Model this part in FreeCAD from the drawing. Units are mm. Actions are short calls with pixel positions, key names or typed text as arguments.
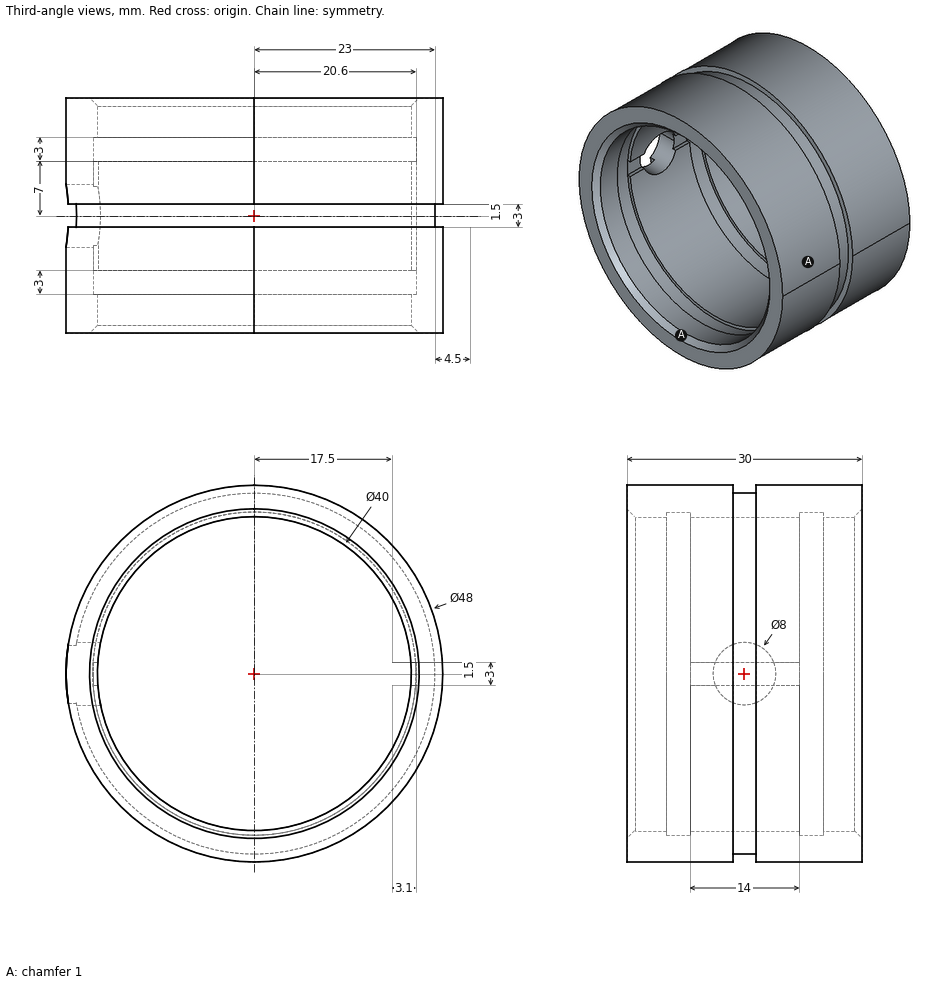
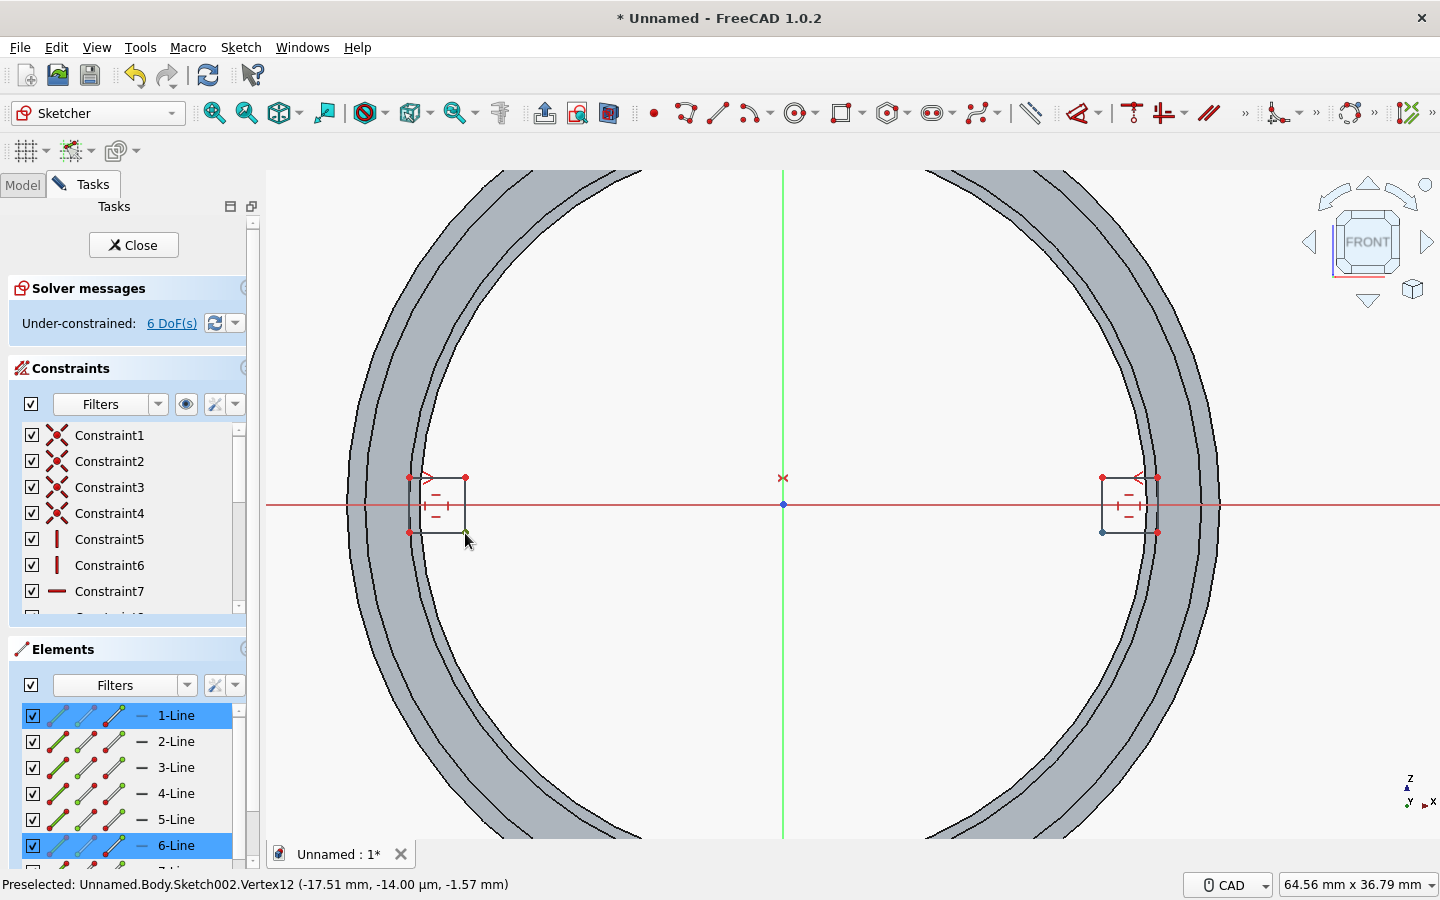
click(783, 767)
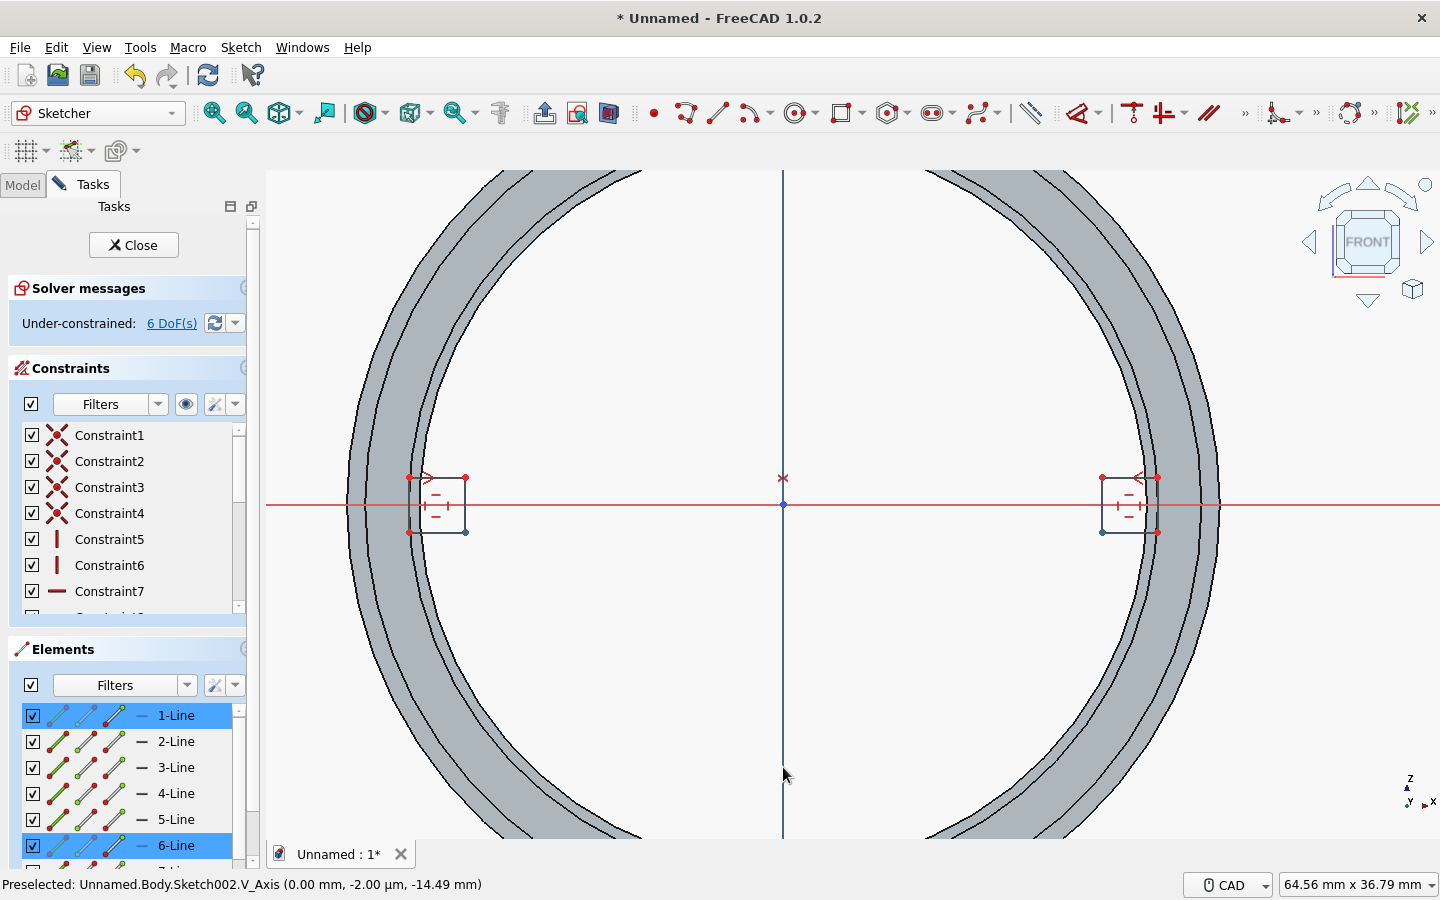
key(s)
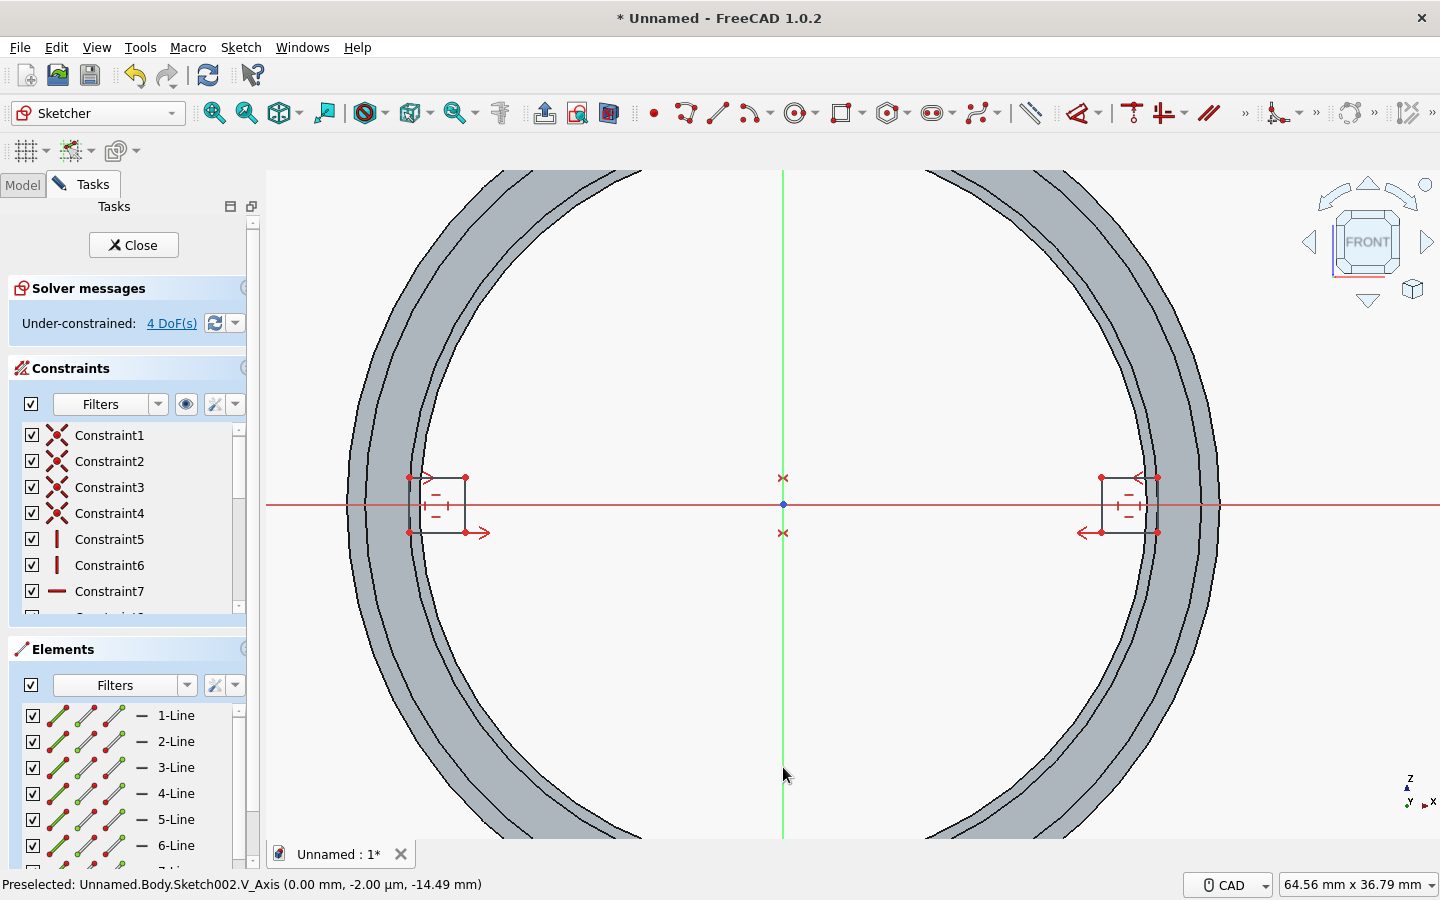
key(d)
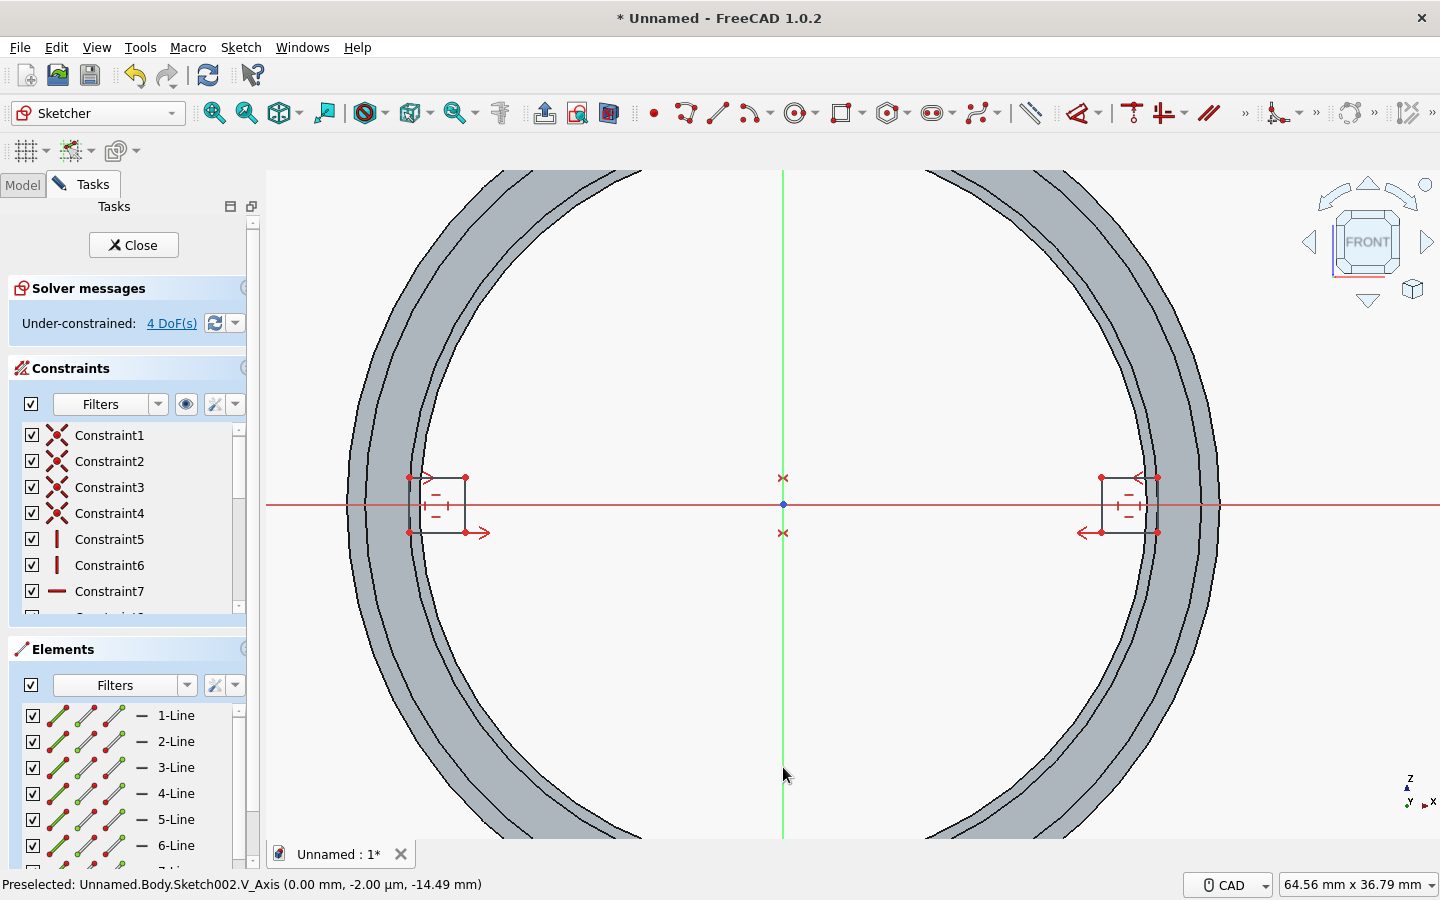
scroll(1102, 495, up, 2)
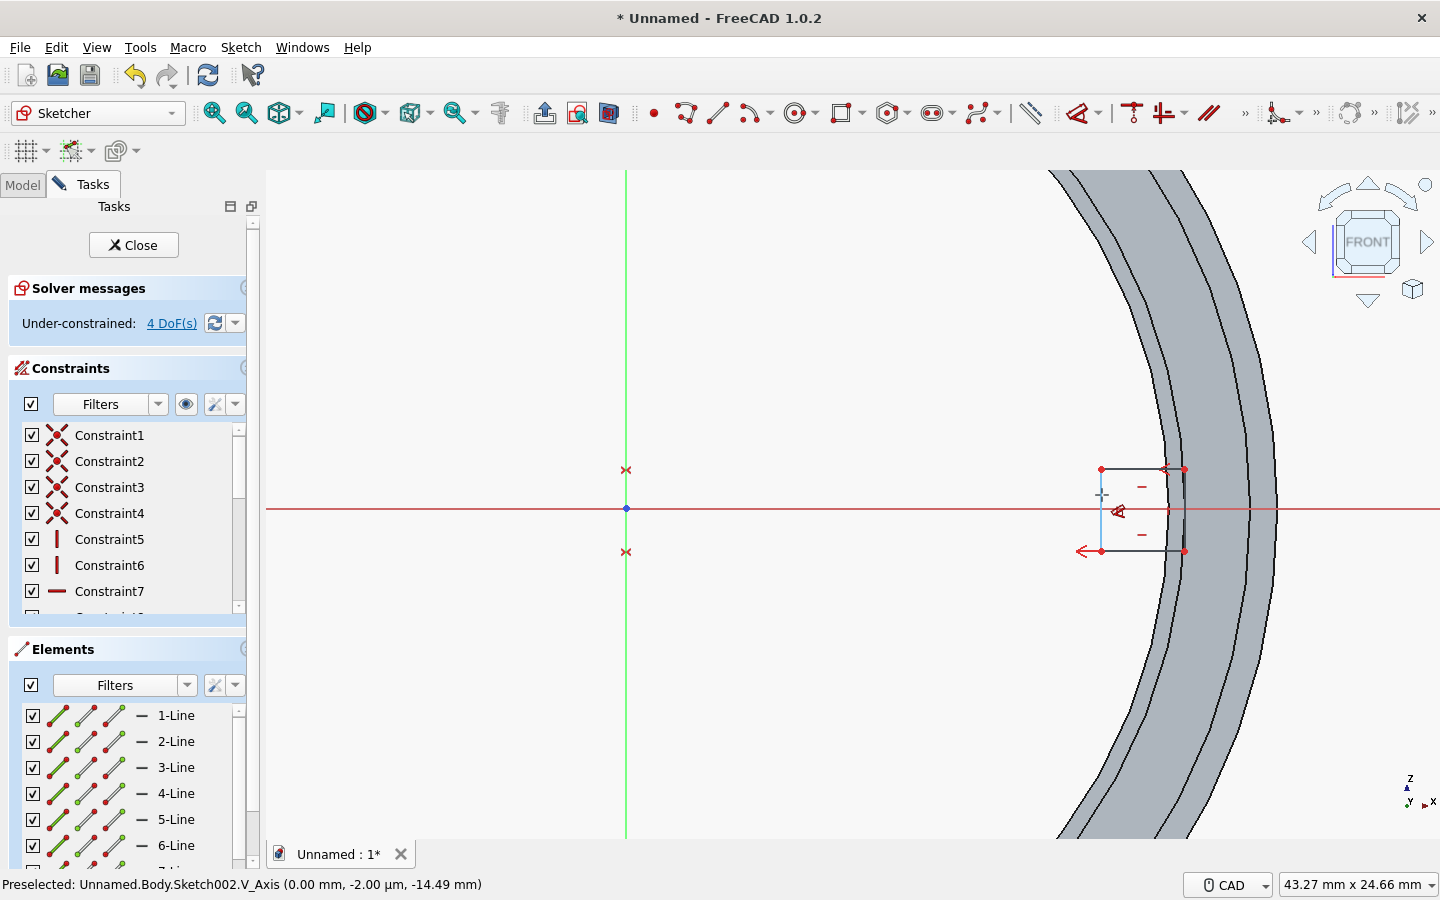
click(1101, 494)
click(1135, 492)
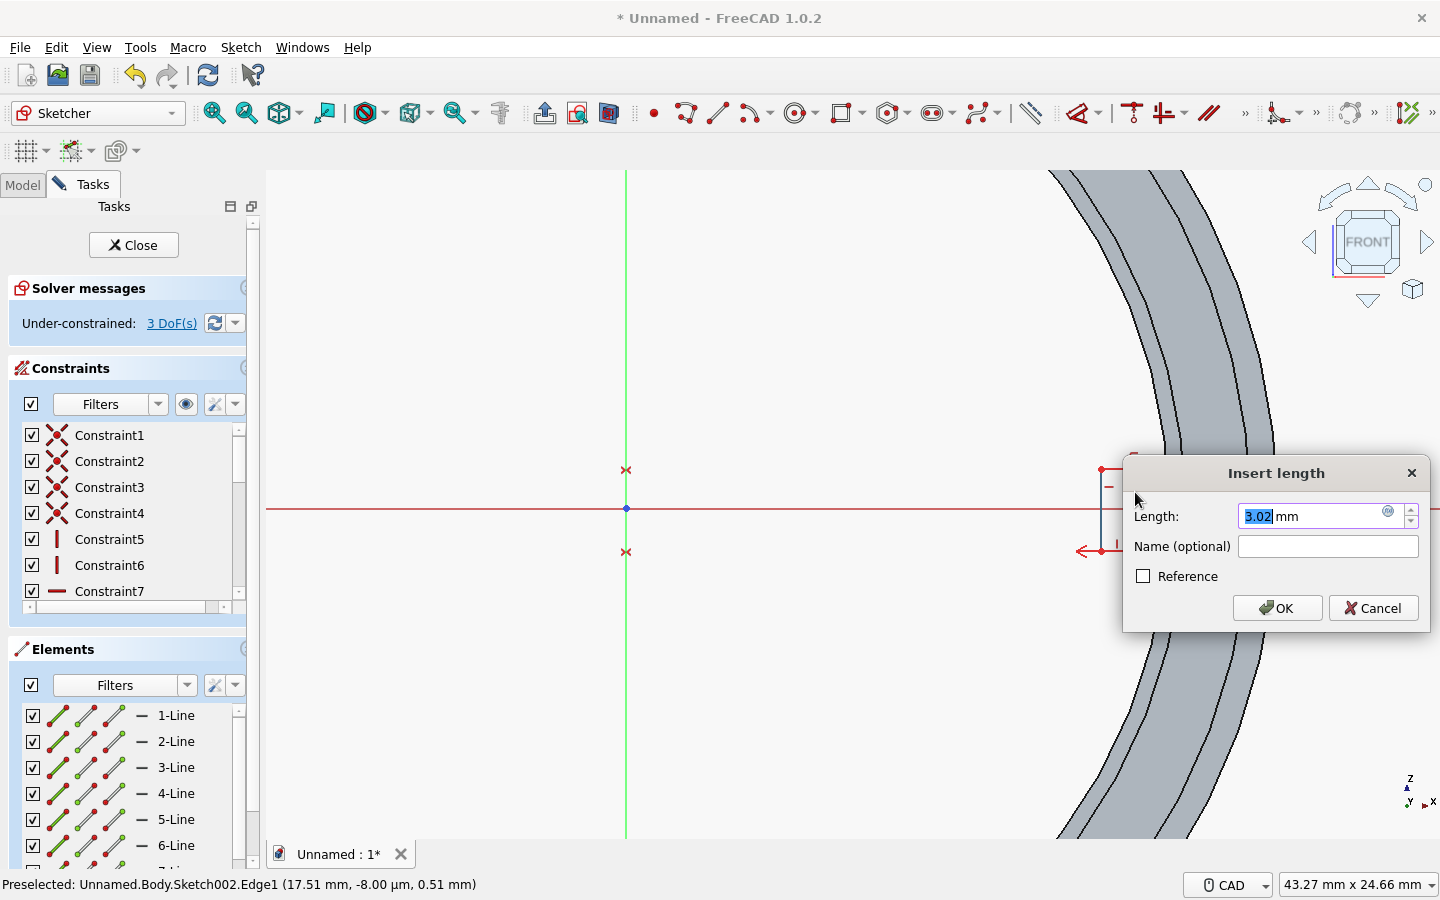
text(3)
key(Return)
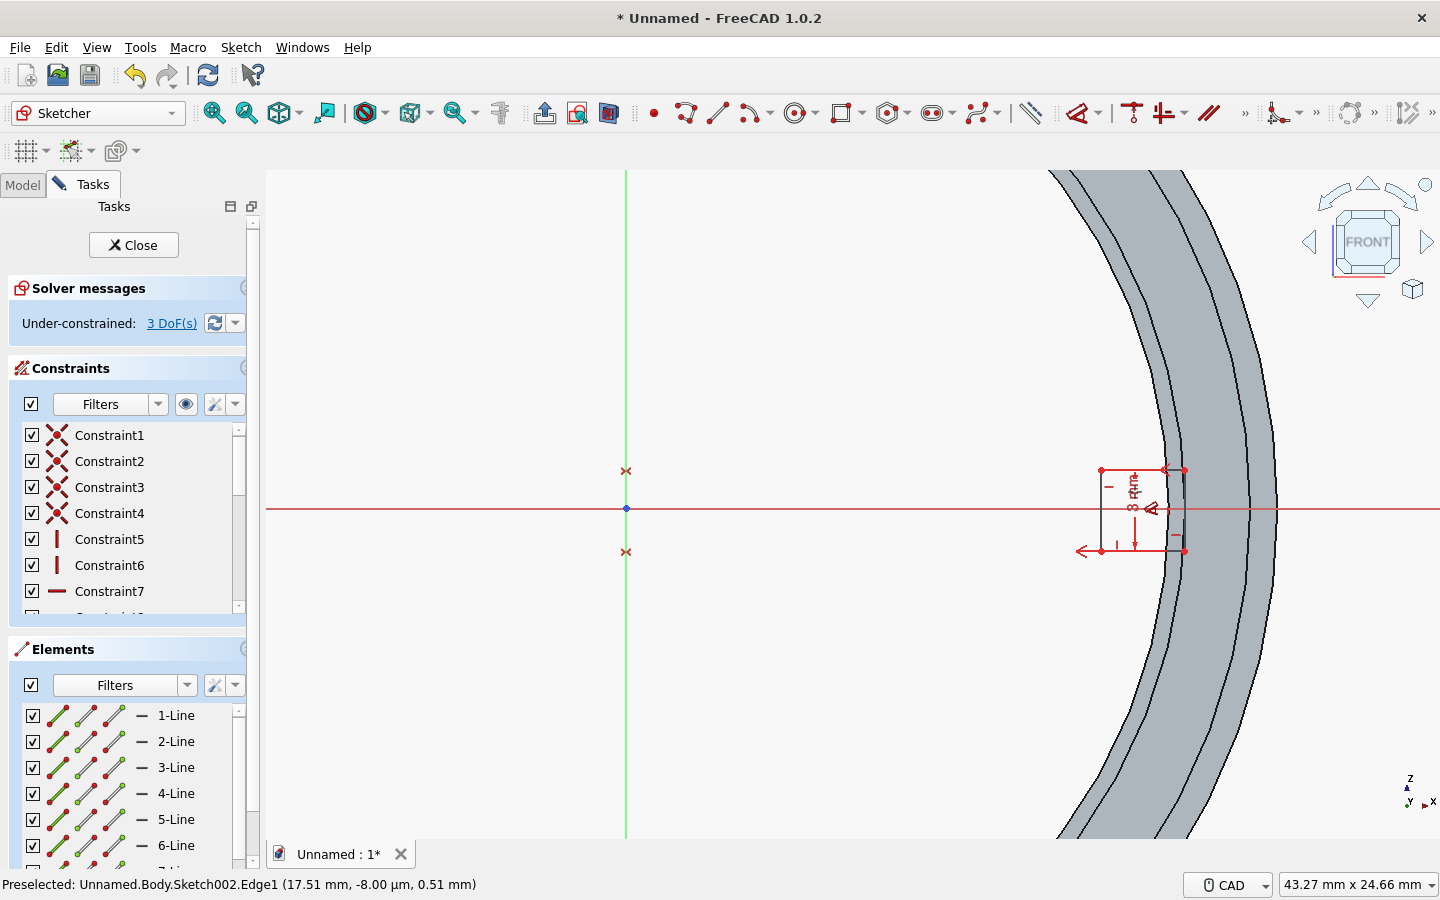
click(1126, 551)
click(1143, 585)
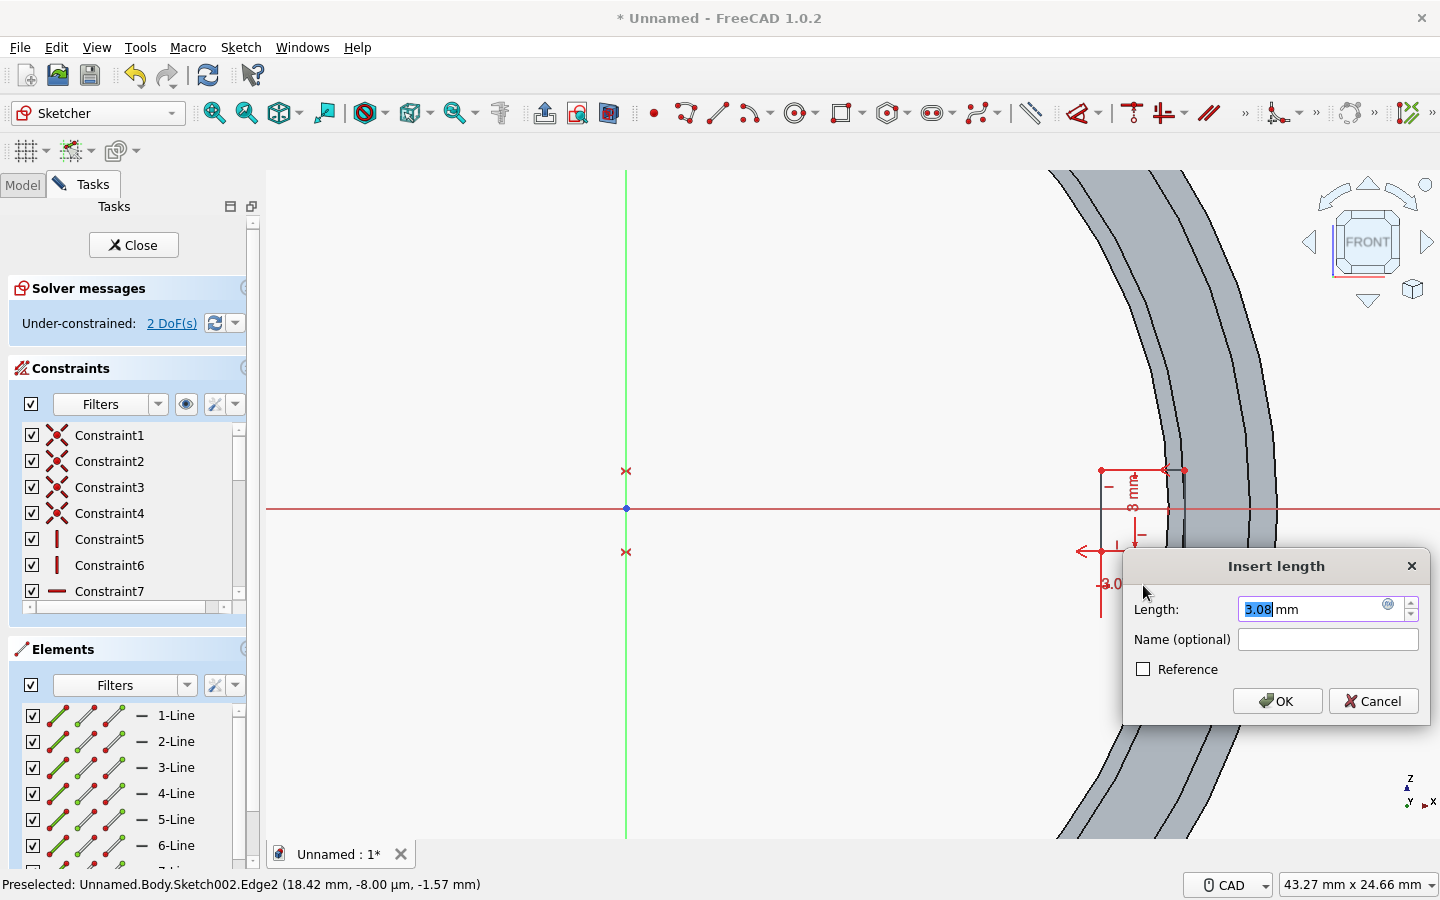
text(3.1)
key(Return)